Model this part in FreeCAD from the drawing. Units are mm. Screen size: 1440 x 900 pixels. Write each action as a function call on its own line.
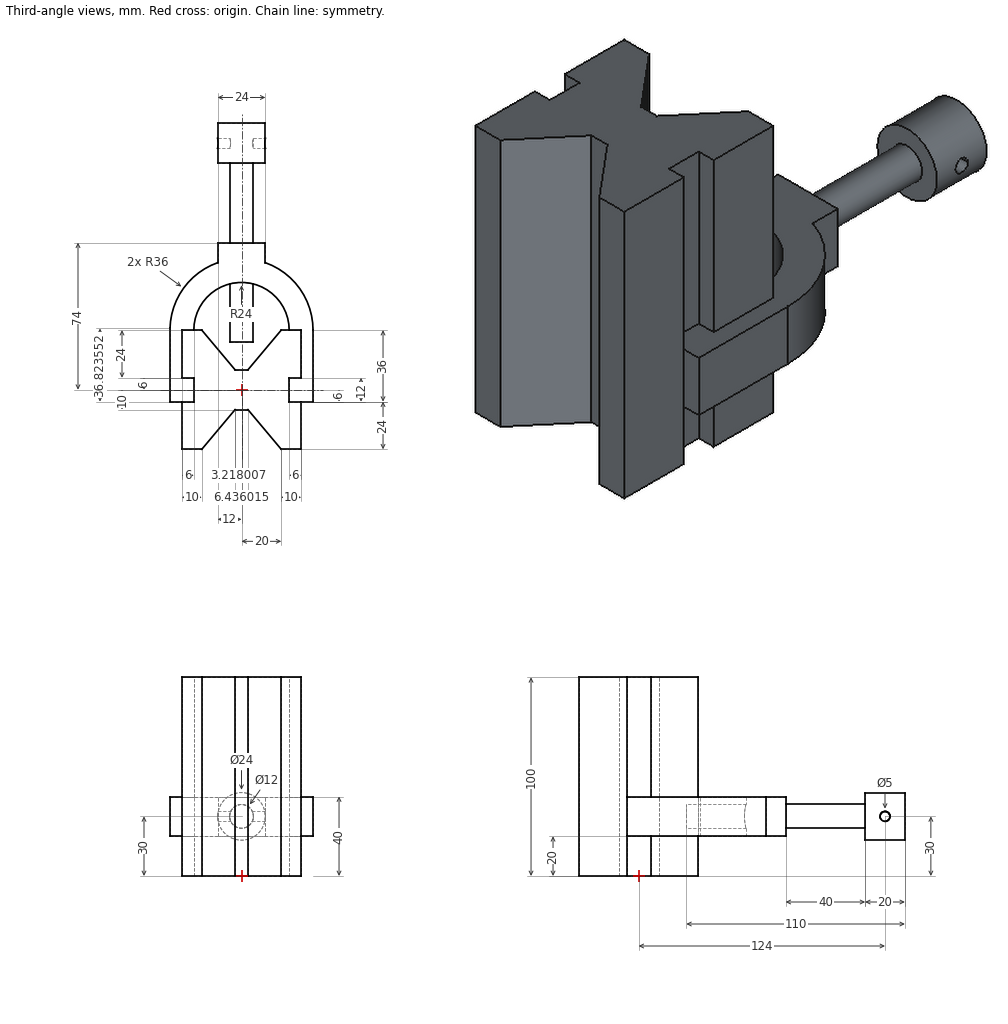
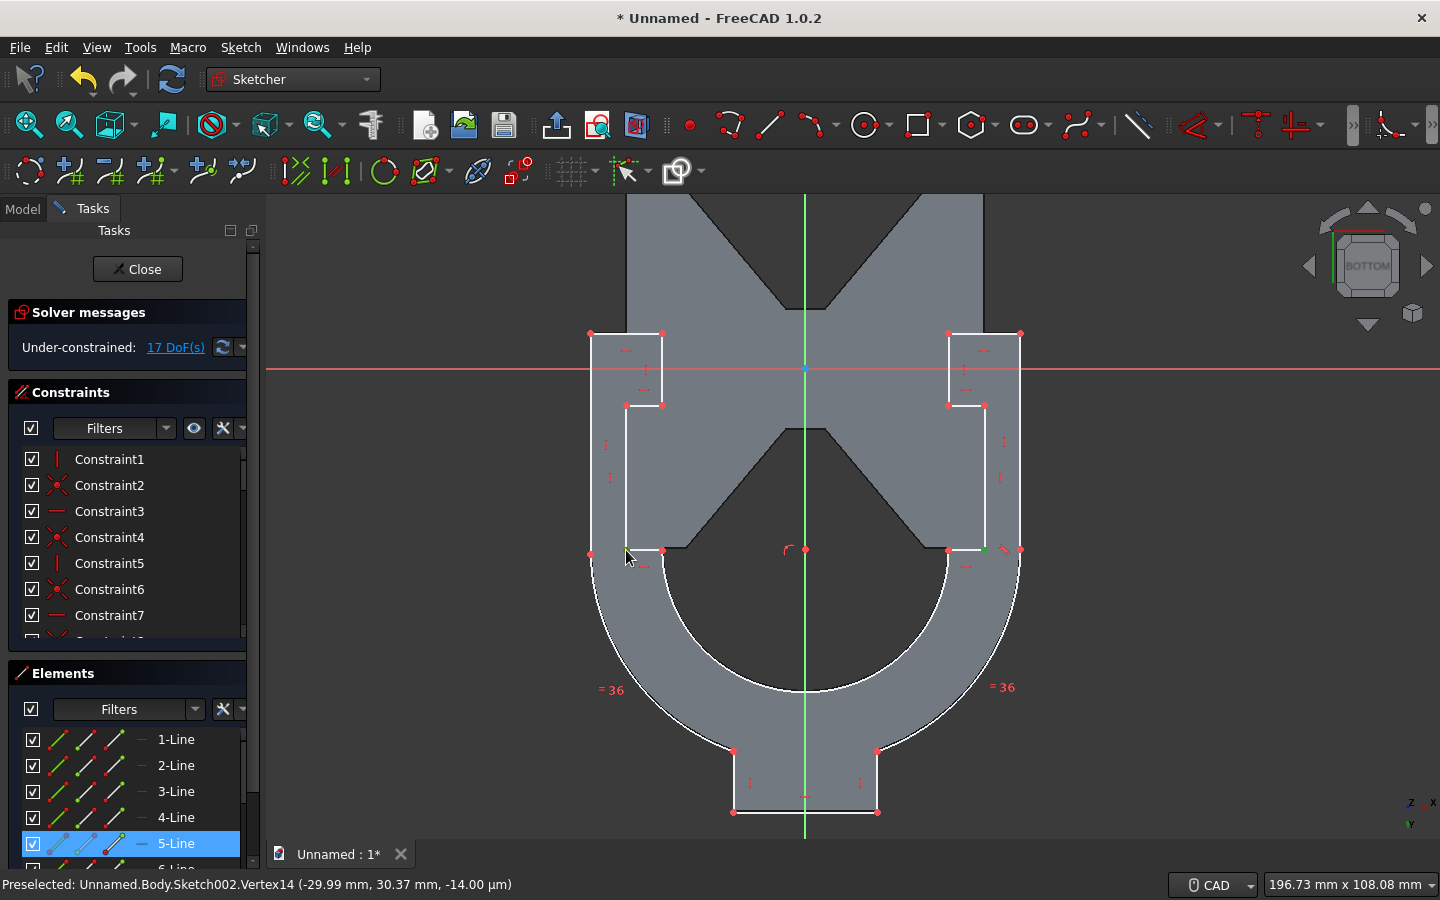
click(805, 769)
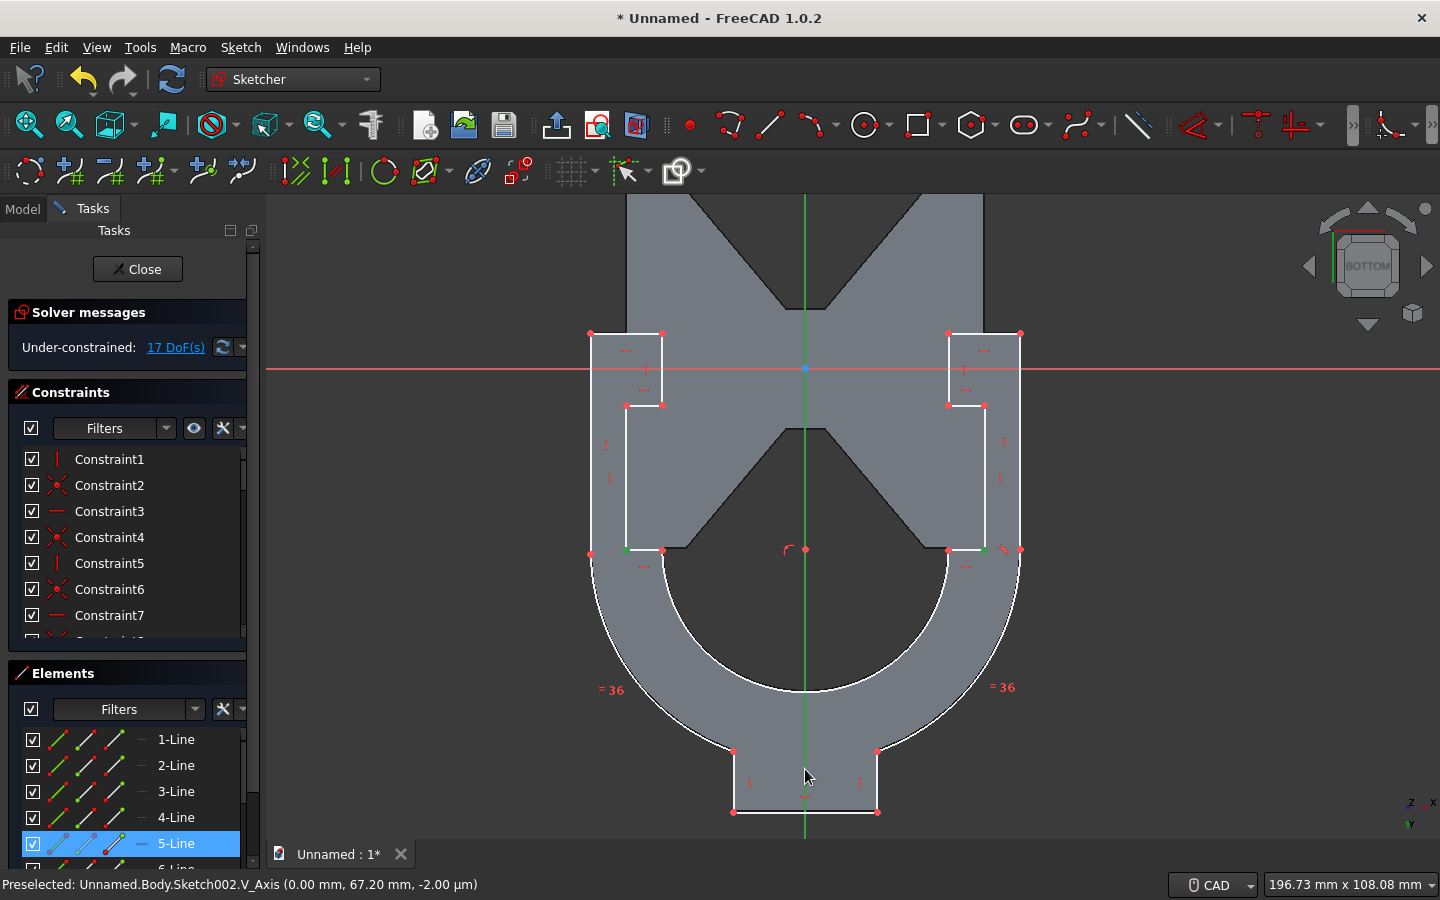
key(s)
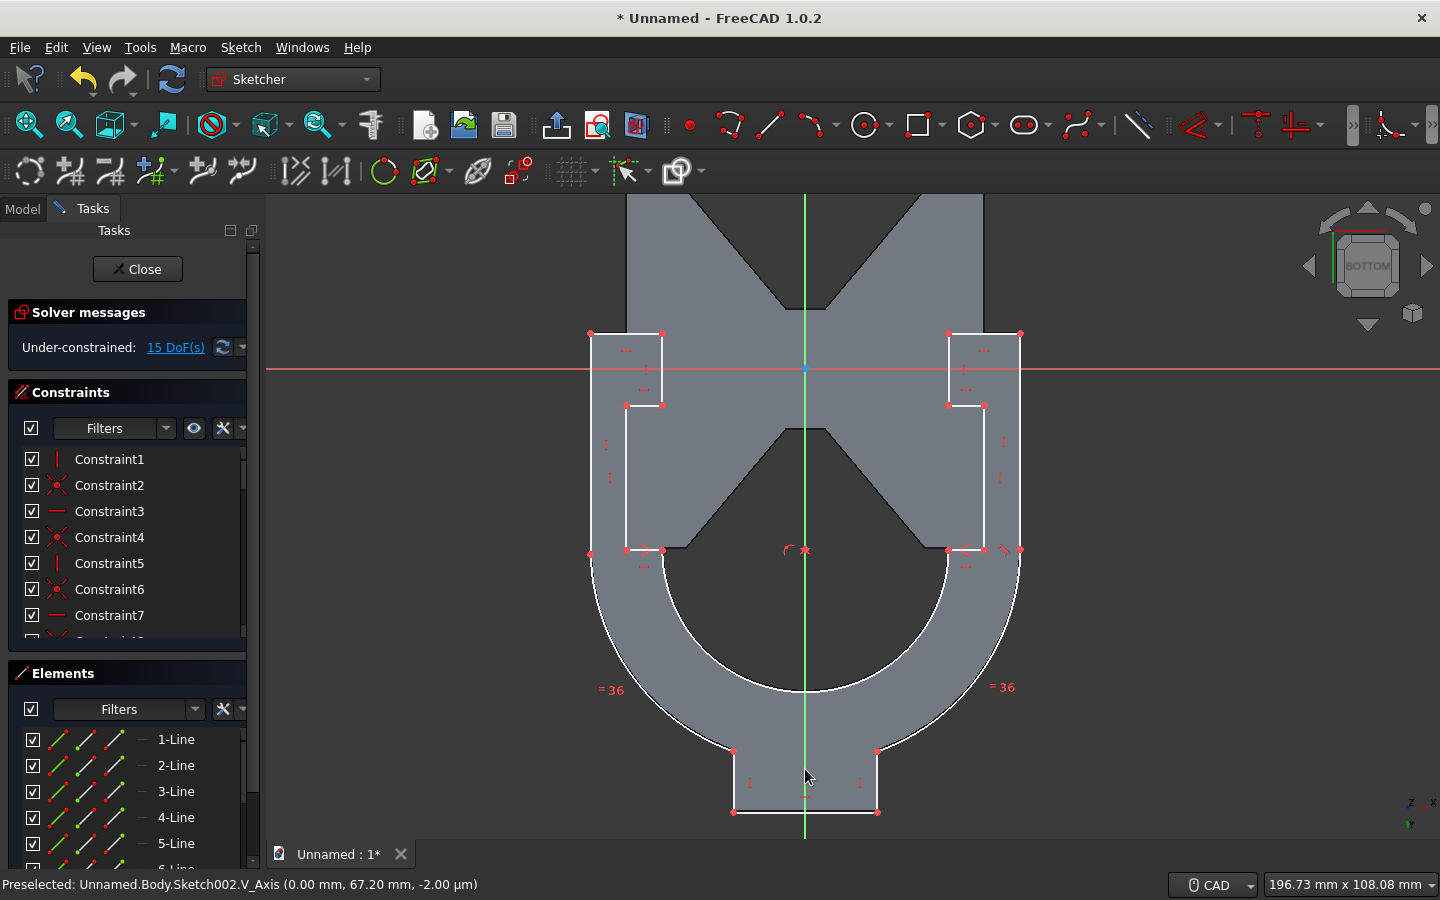
click(949, 406)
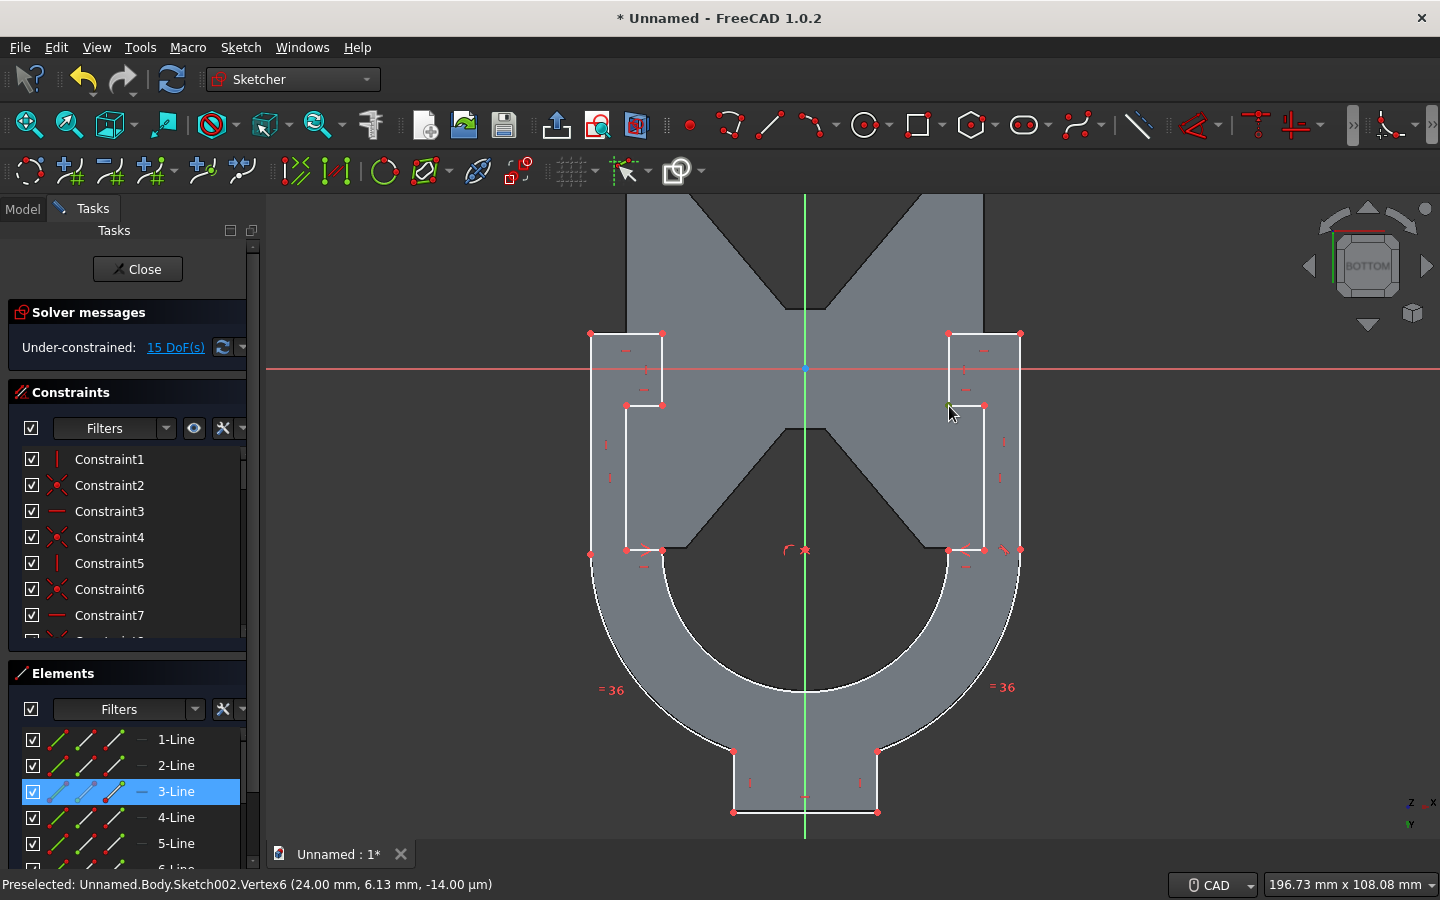
click(662, 406)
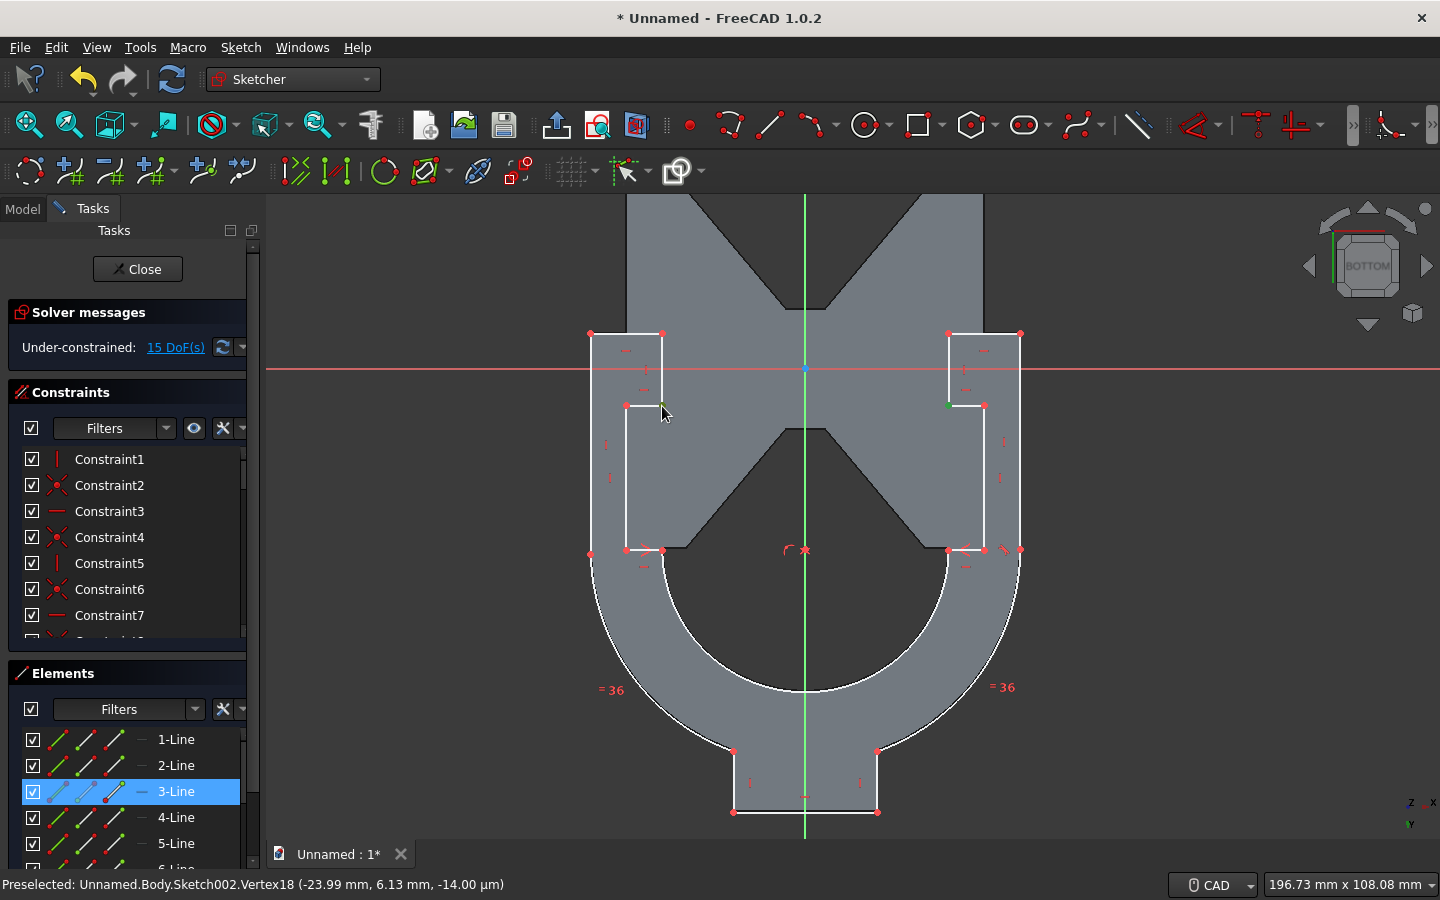
click(805, 769)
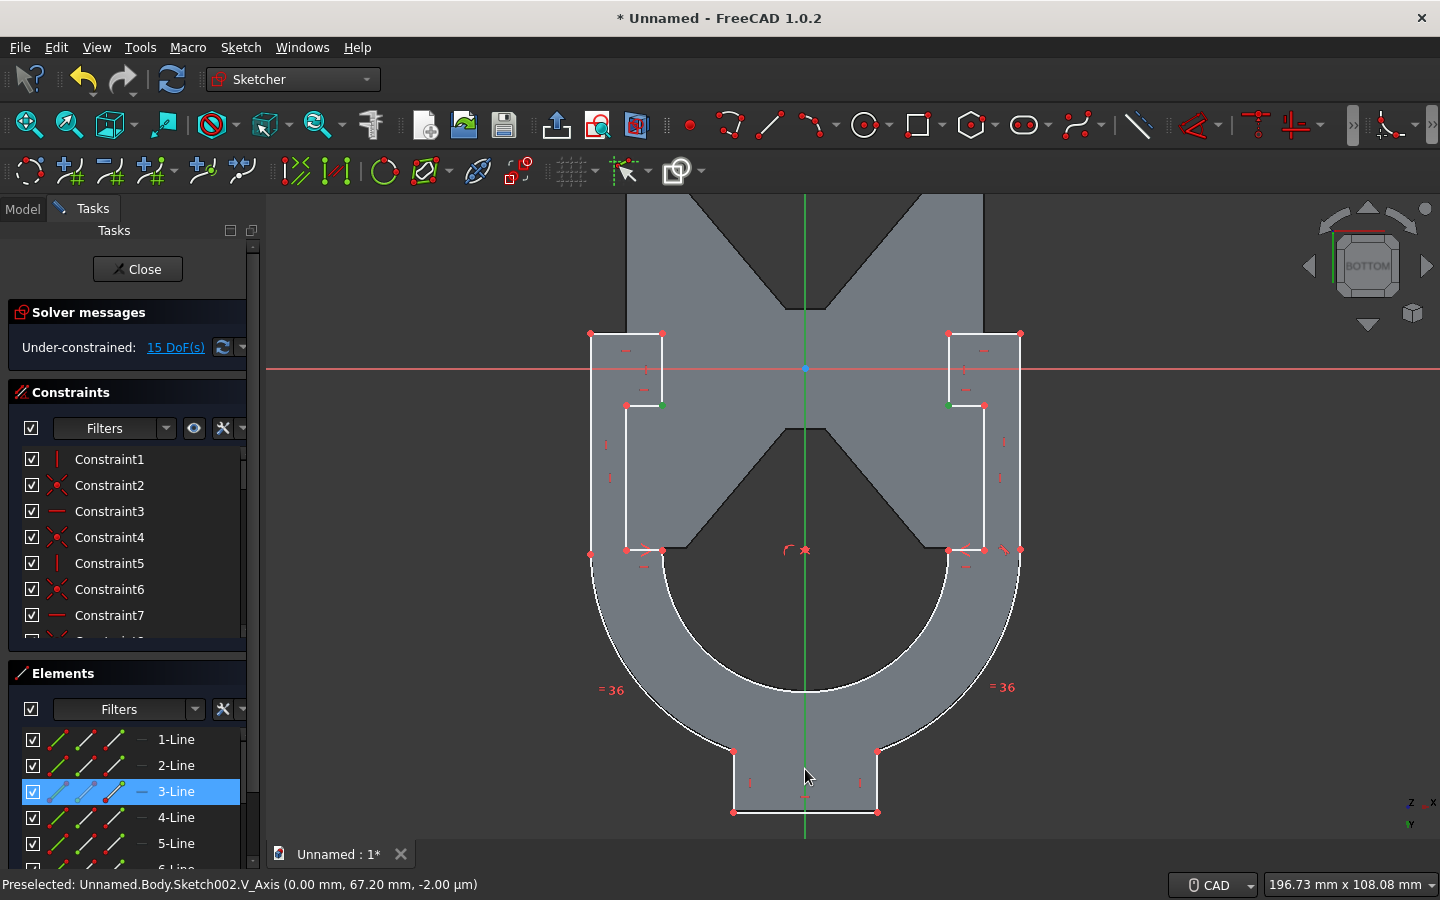
key(s)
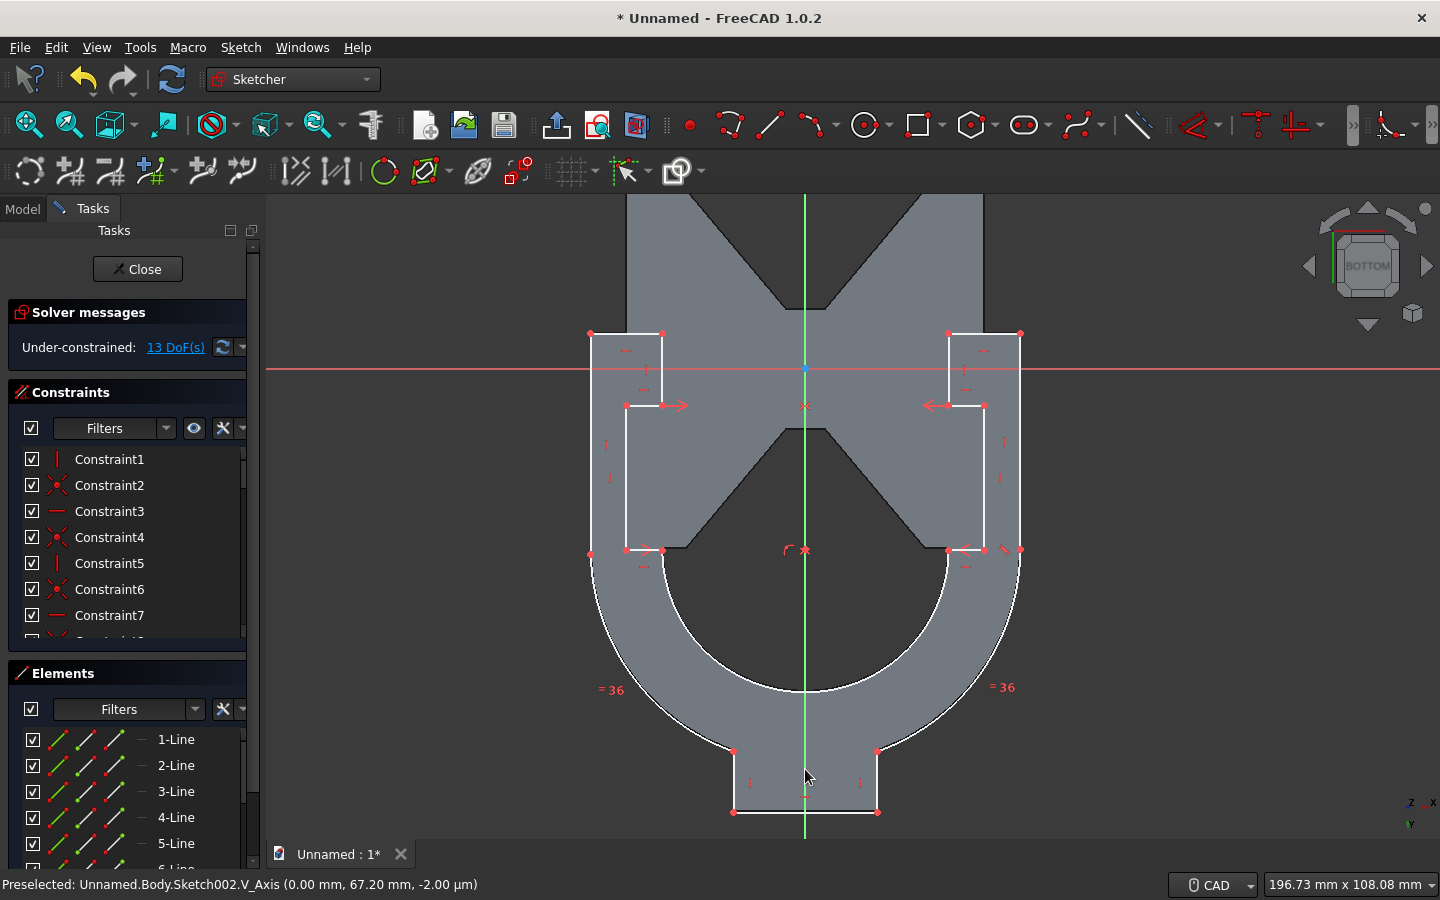
key(d)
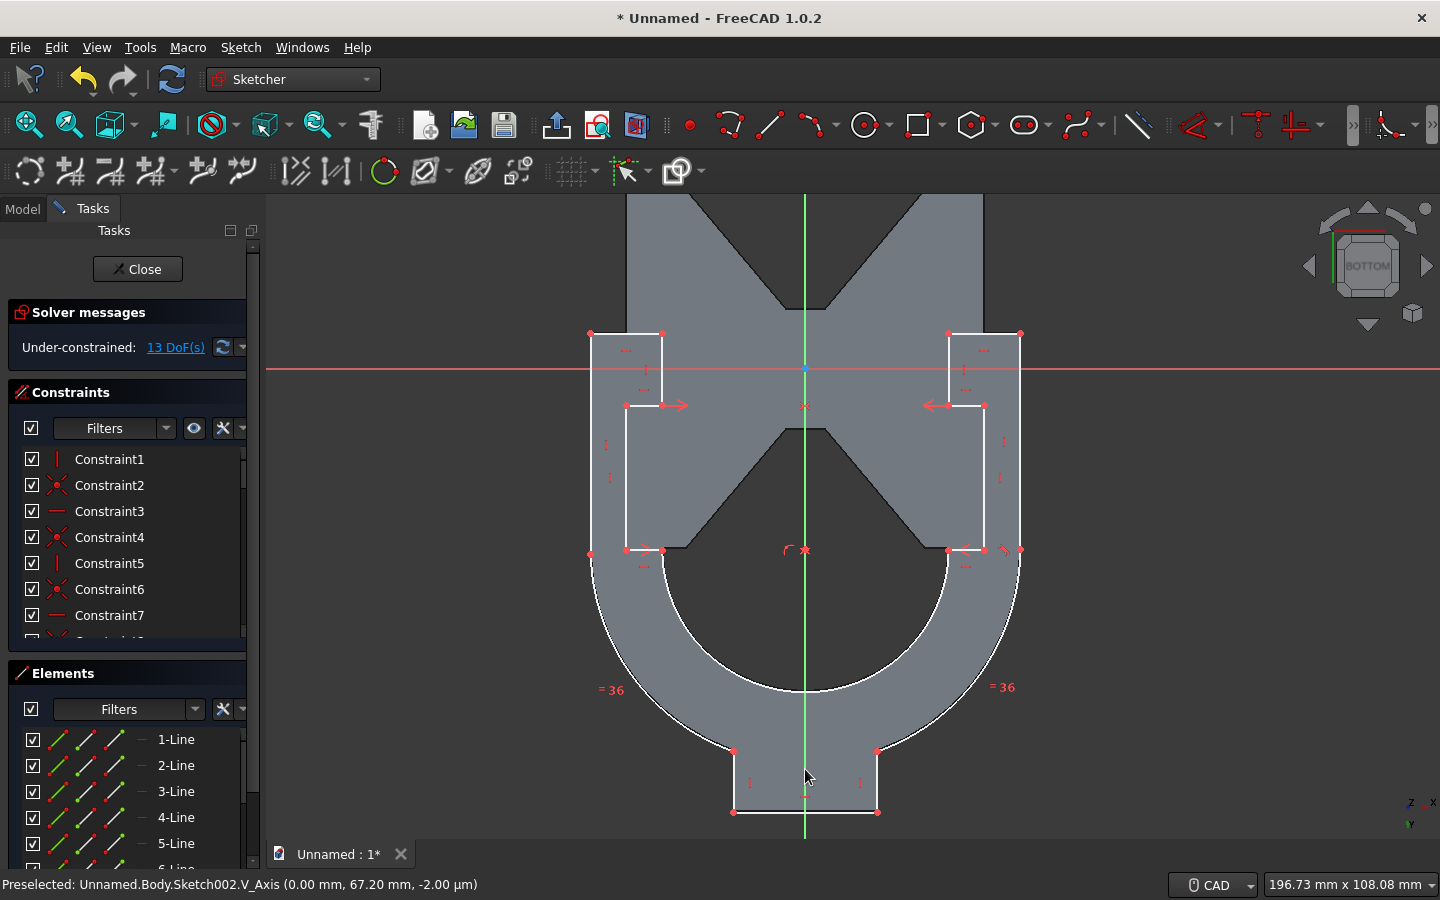
click(722, 665)
click(703, 691)